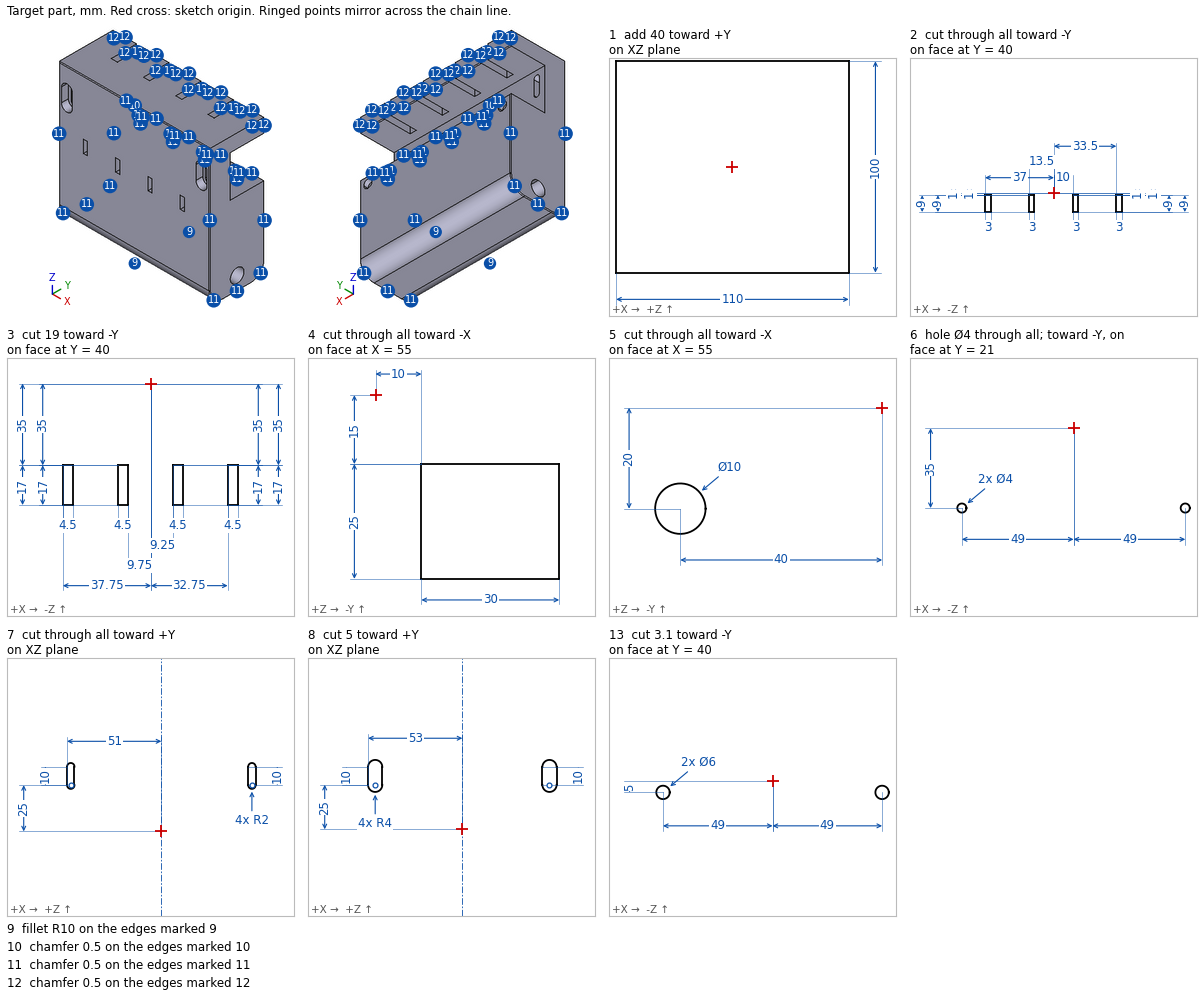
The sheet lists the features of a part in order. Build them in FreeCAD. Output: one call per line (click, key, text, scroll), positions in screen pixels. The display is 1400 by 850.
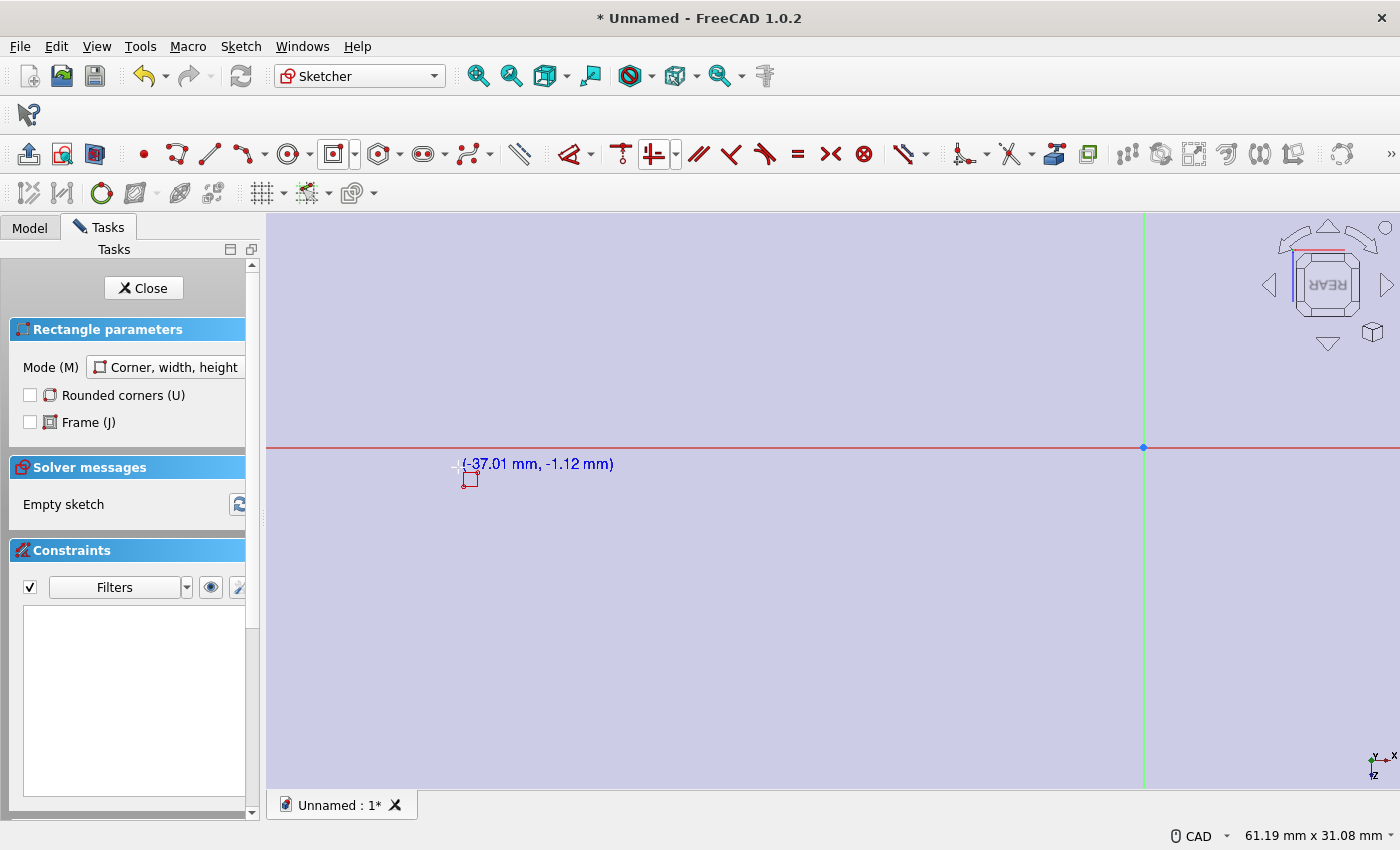
click(458, 466)
click(514, 633)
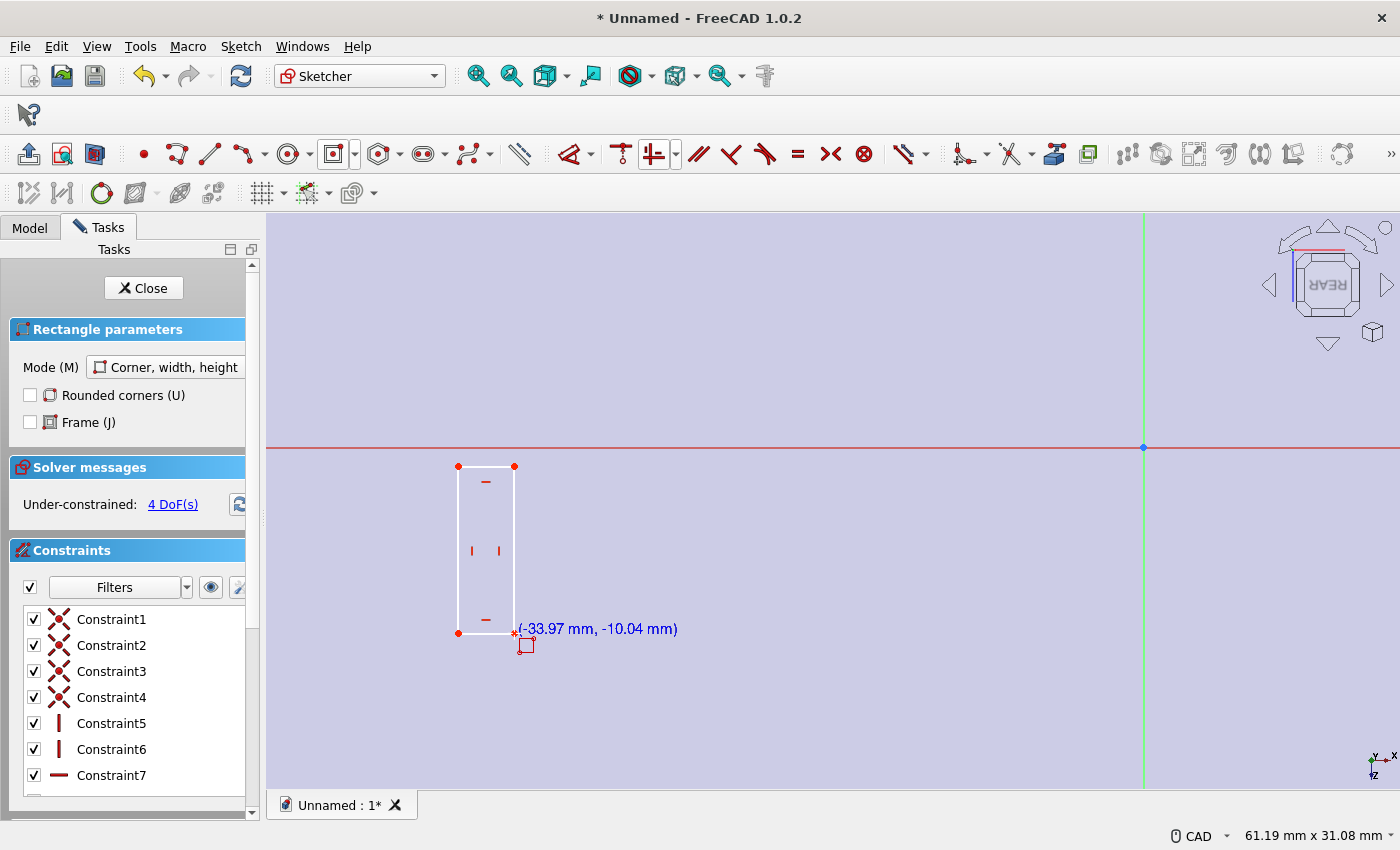
click(893, 466)
click(949, 633)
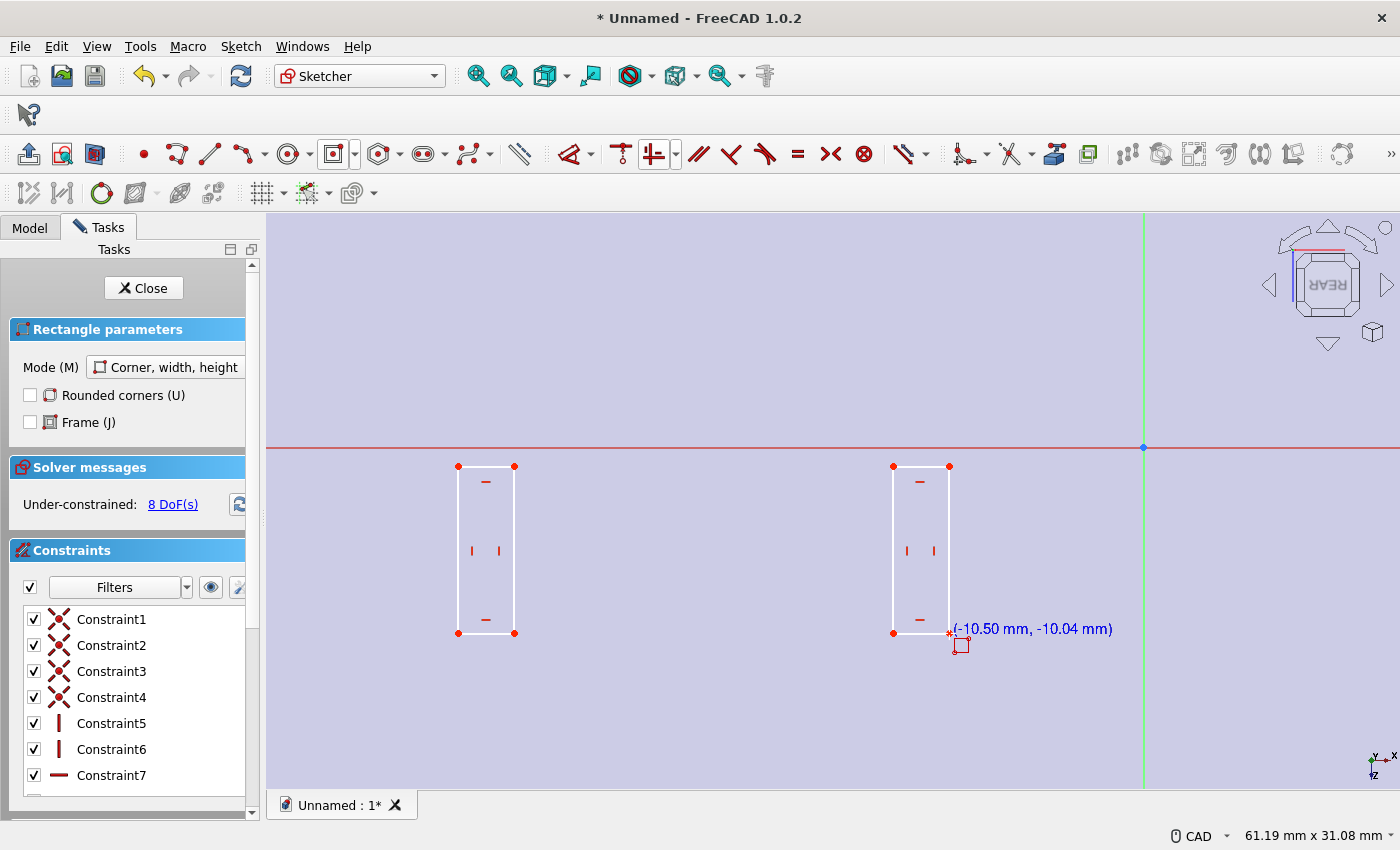
scroll(459, 469, down, 4)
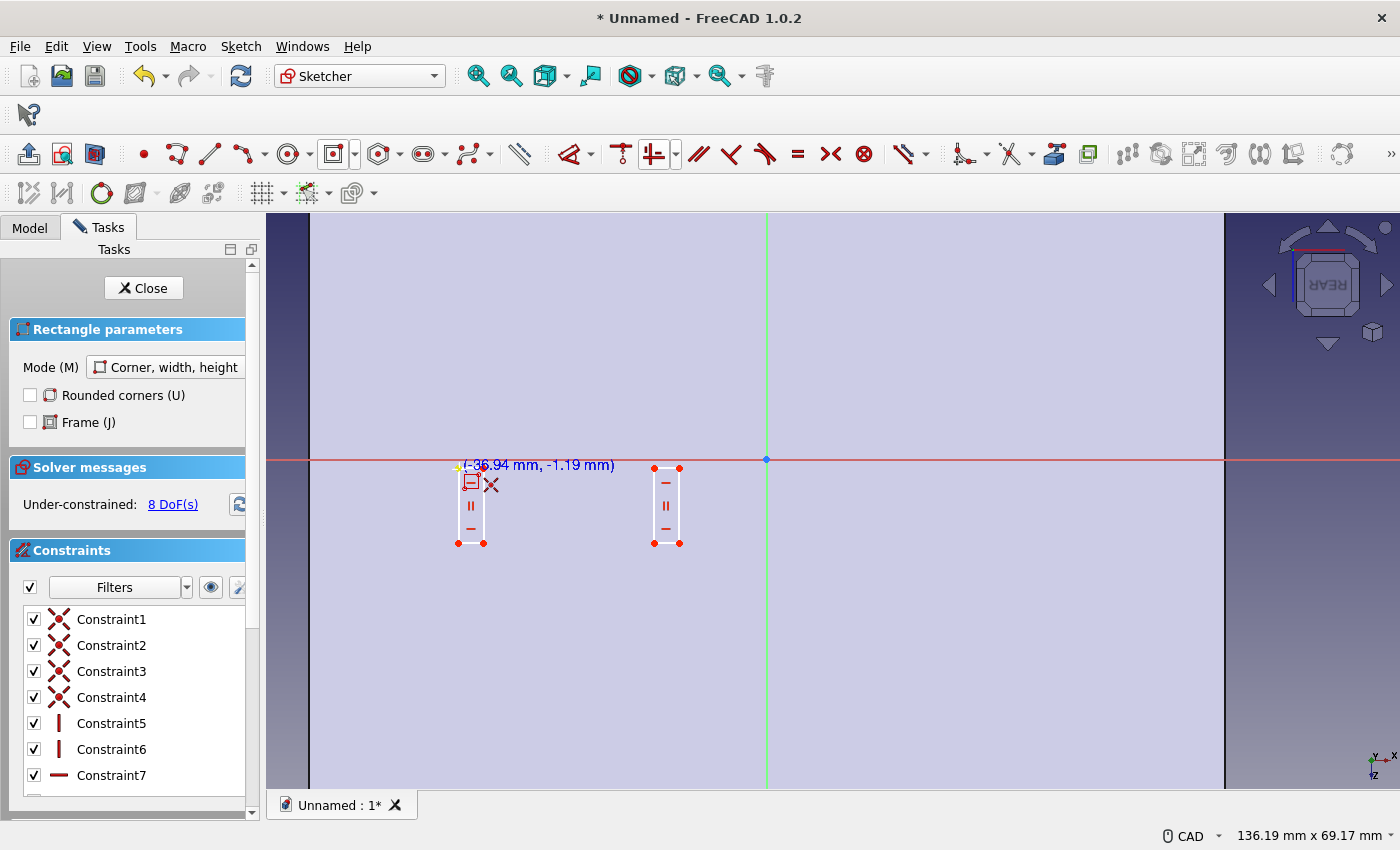
scroll(850, 468, up, 4)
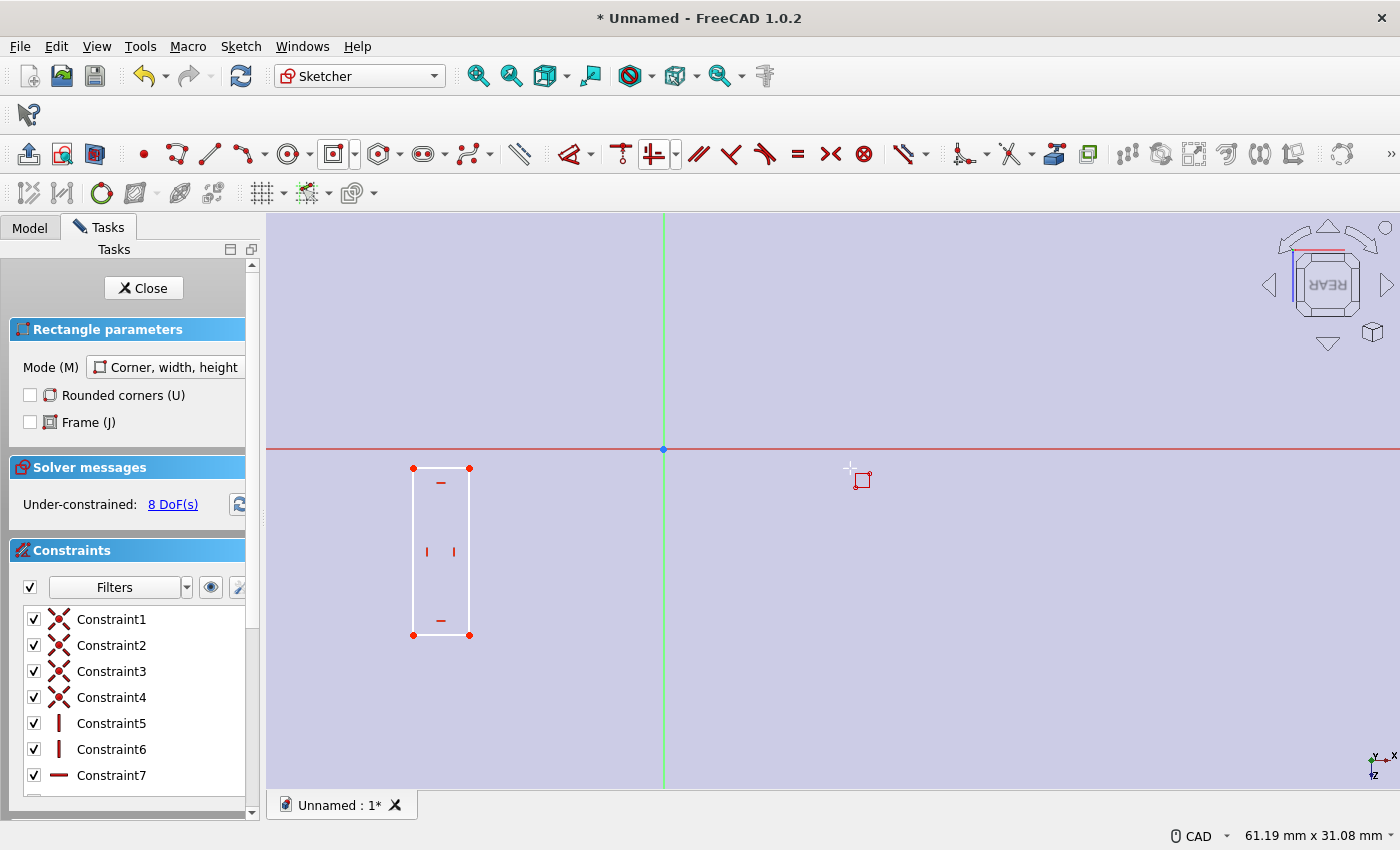
click(849, 468)
click(905, 634)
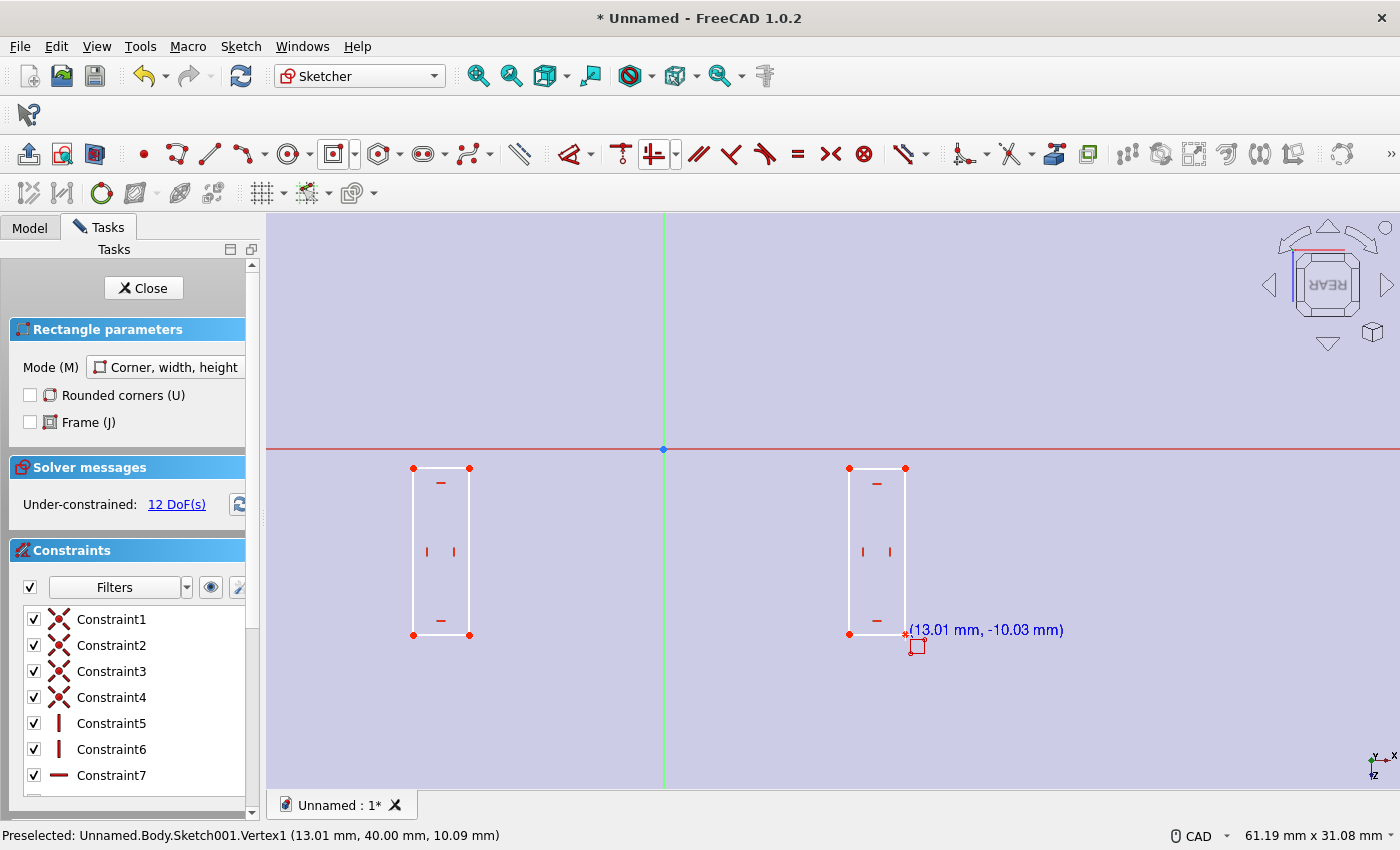
scroll(850, 468, down, 4)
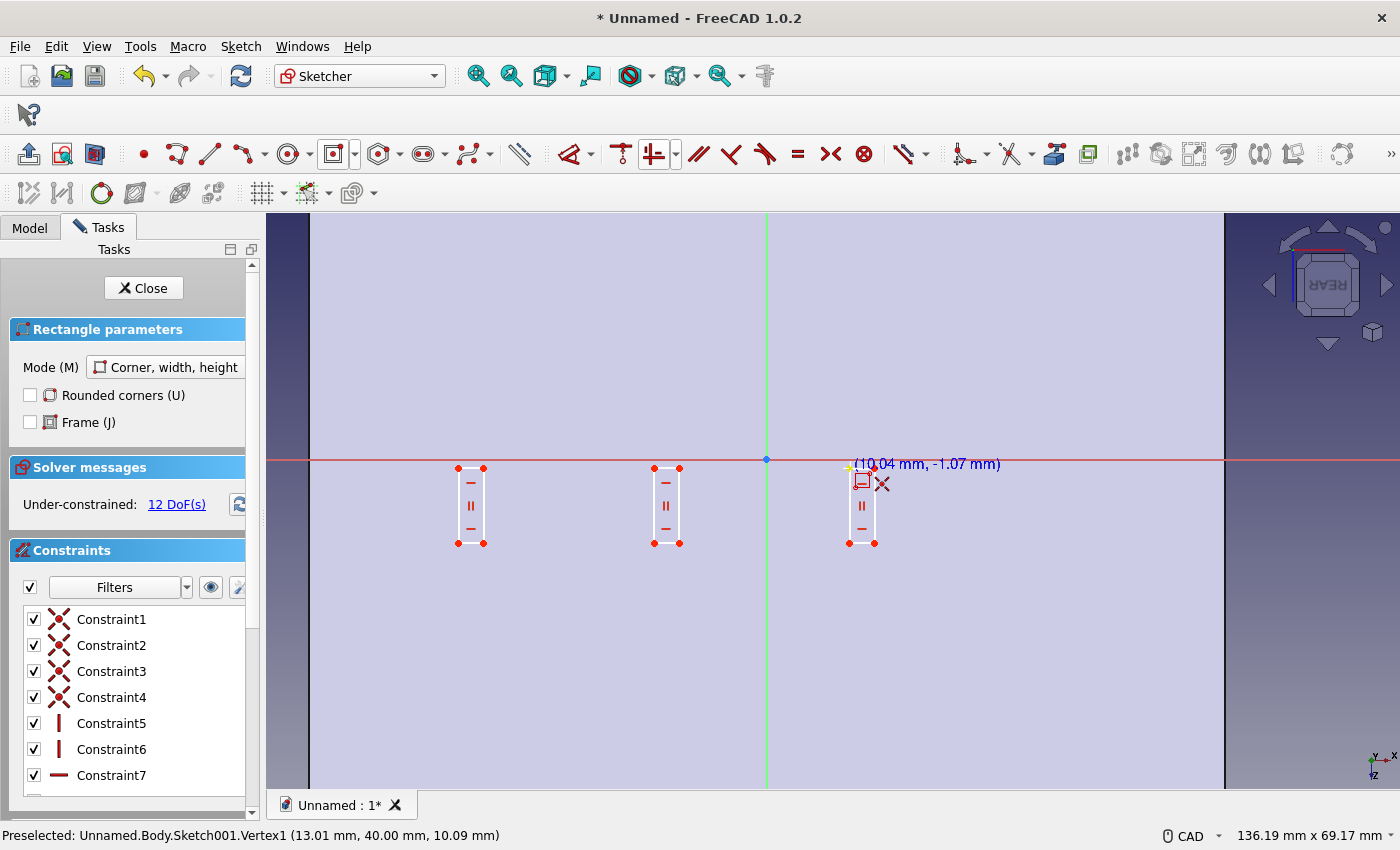
scroll(1046, 468, up, 4)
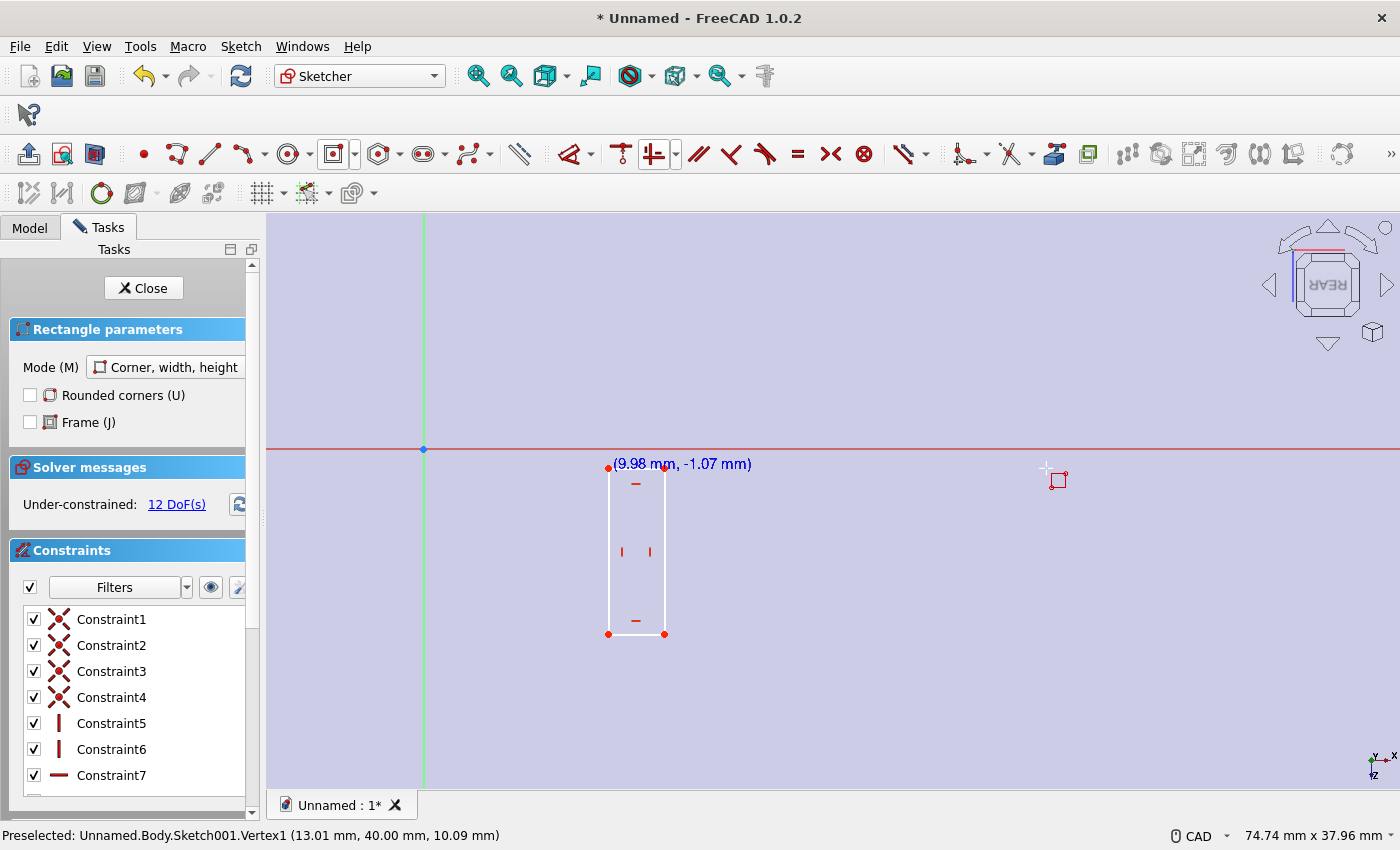
click(1044, 468)
click(1100, 634)
key(Escape)